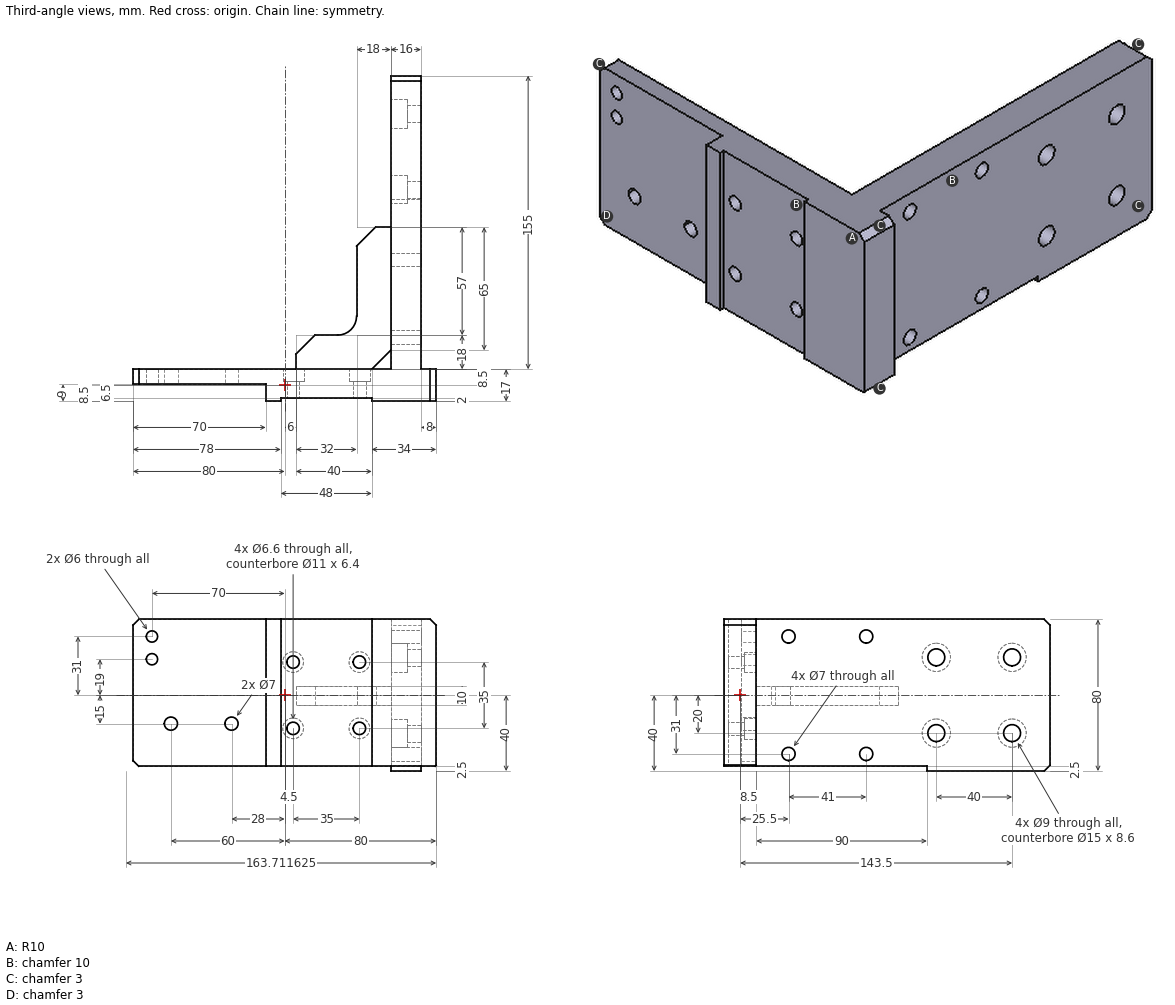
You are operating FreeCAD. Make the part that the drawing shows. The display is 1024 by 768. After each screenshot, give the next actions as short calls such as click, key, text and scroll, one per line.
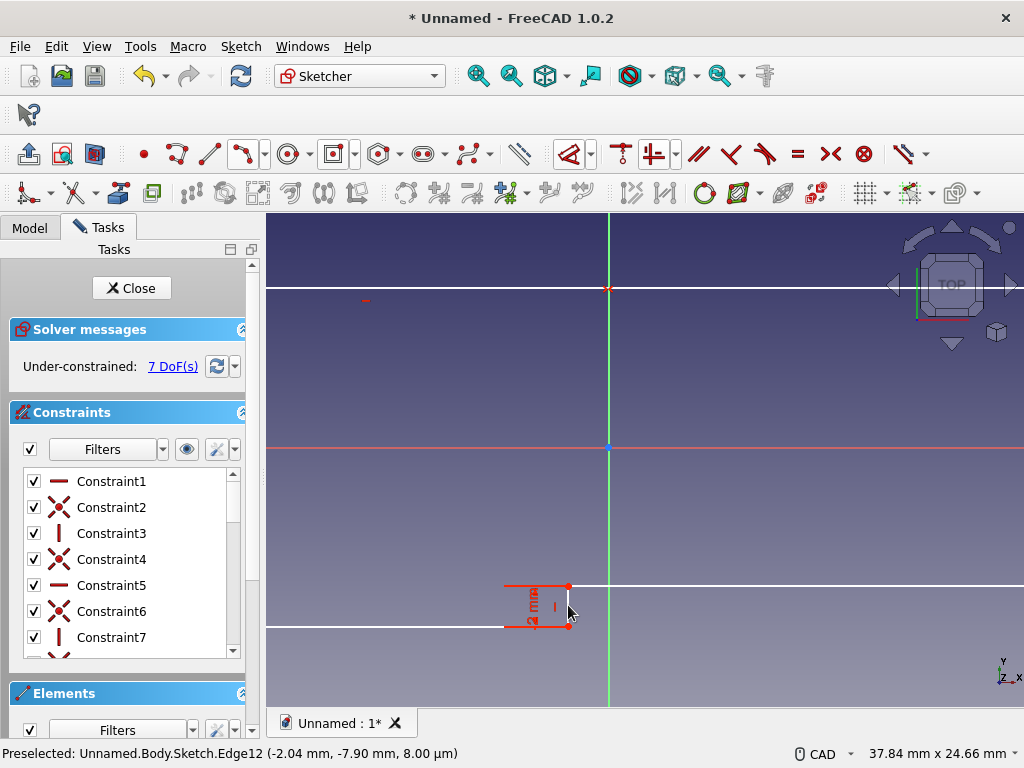
scroll(573, 616, down, 12)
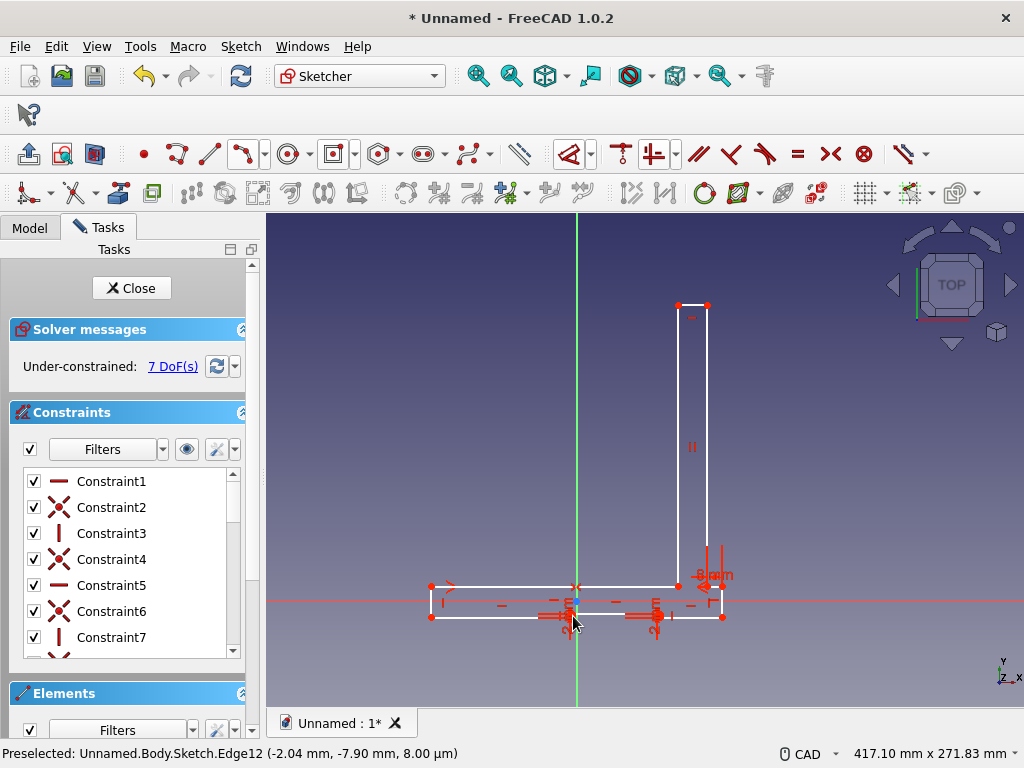
click(599, 614)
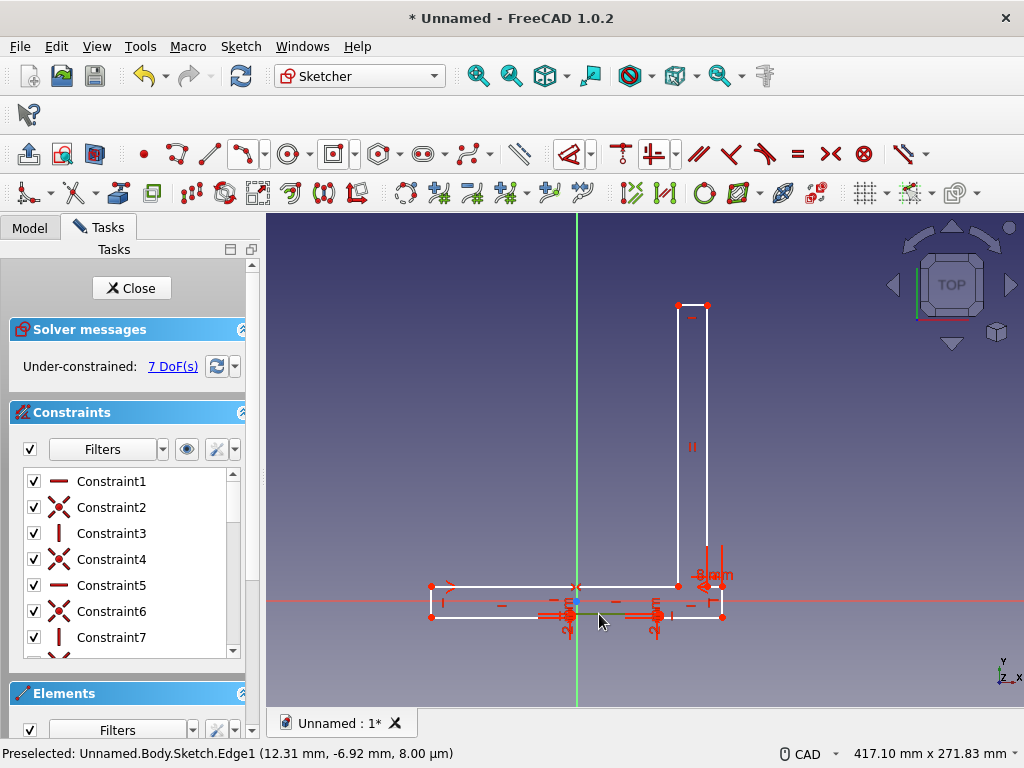
click(590, 154)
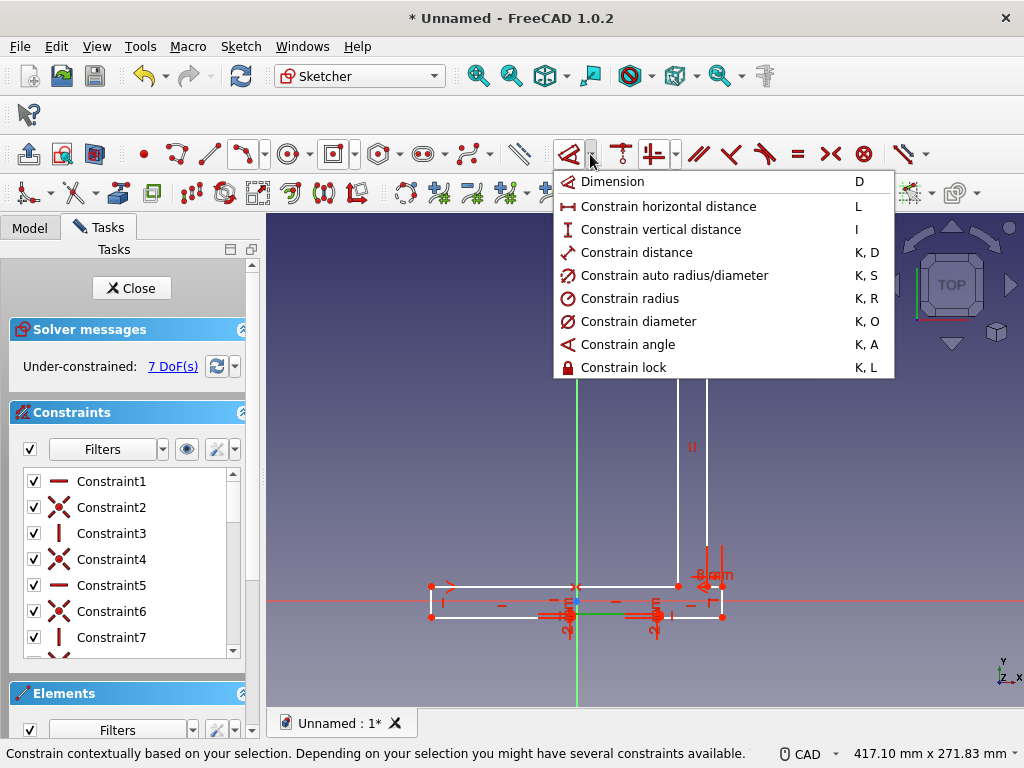
click(724, 206)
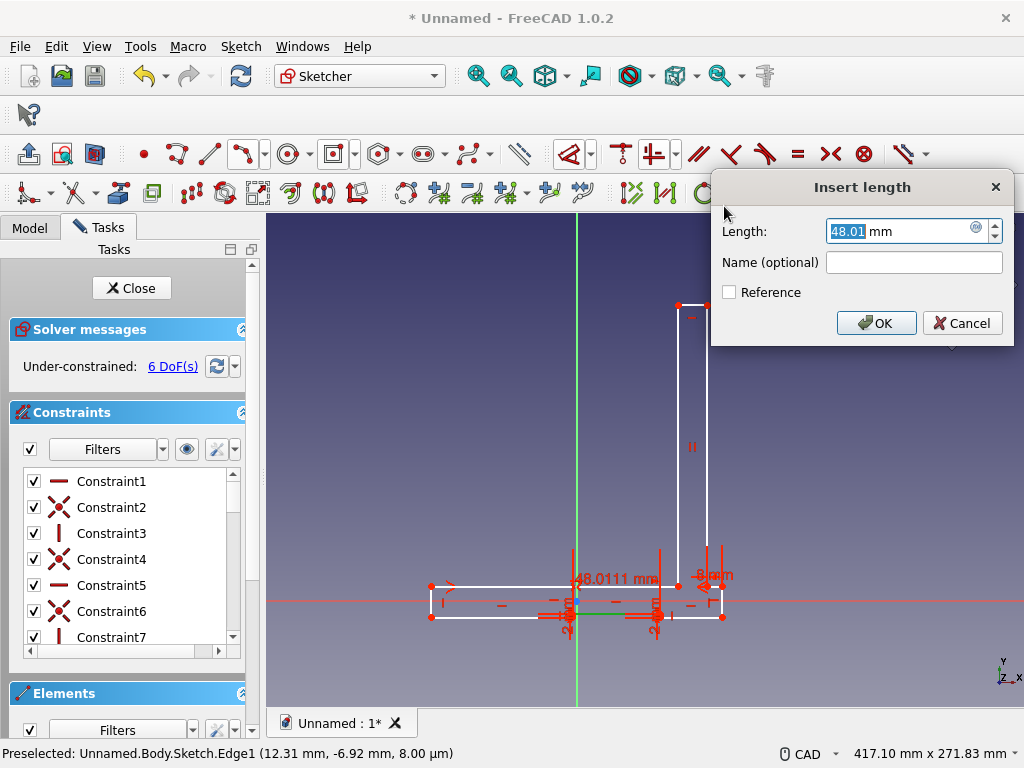
text(48)
key(Return)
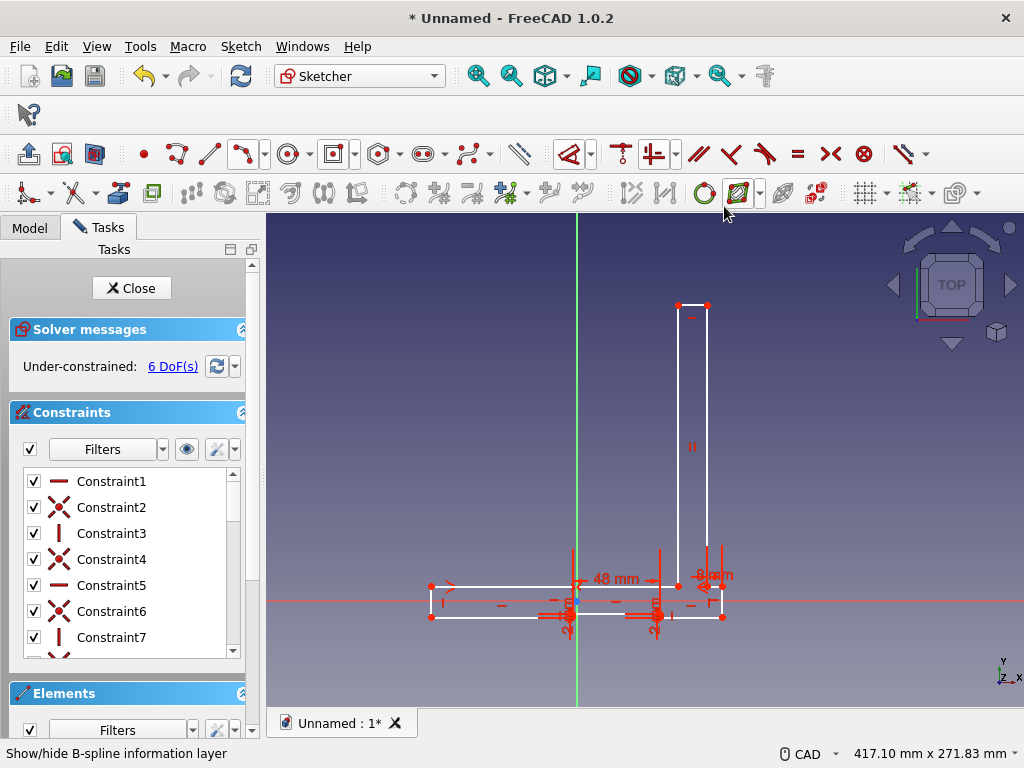
click(679, 618)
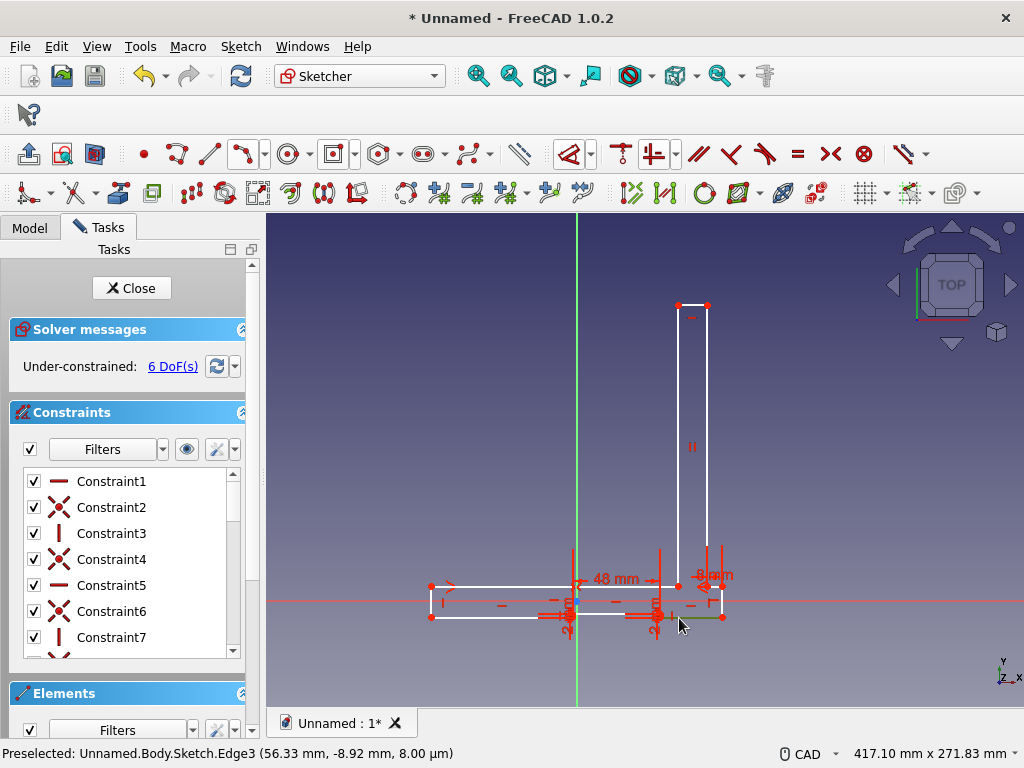
click(590, 154)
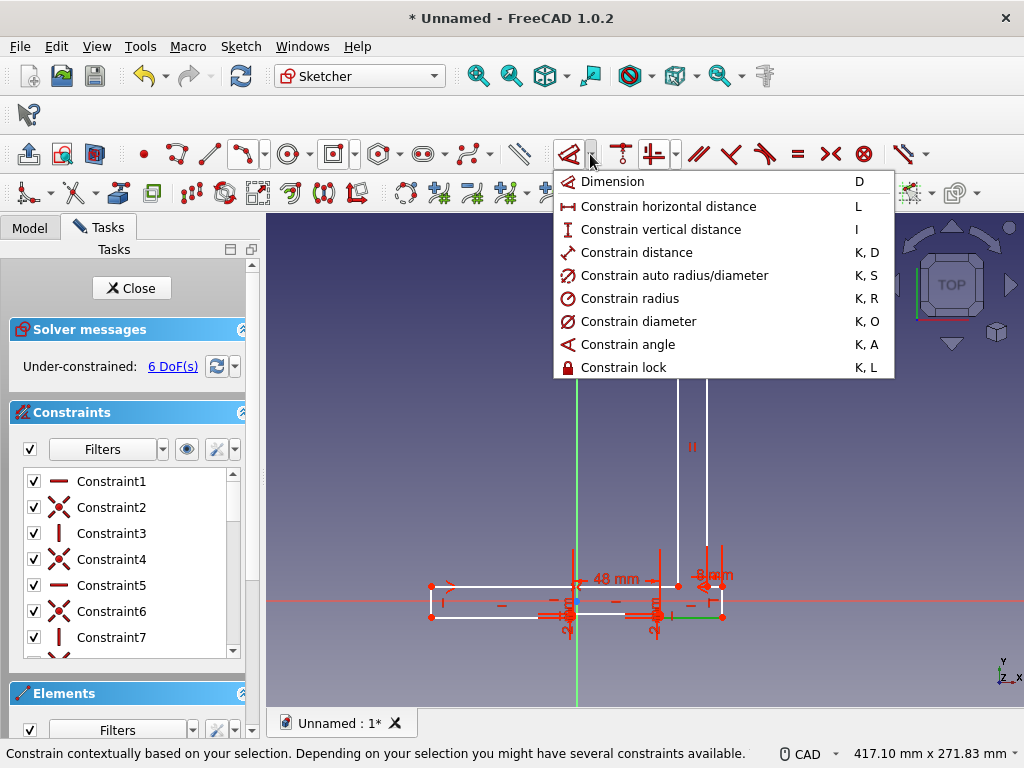
click(724, 206)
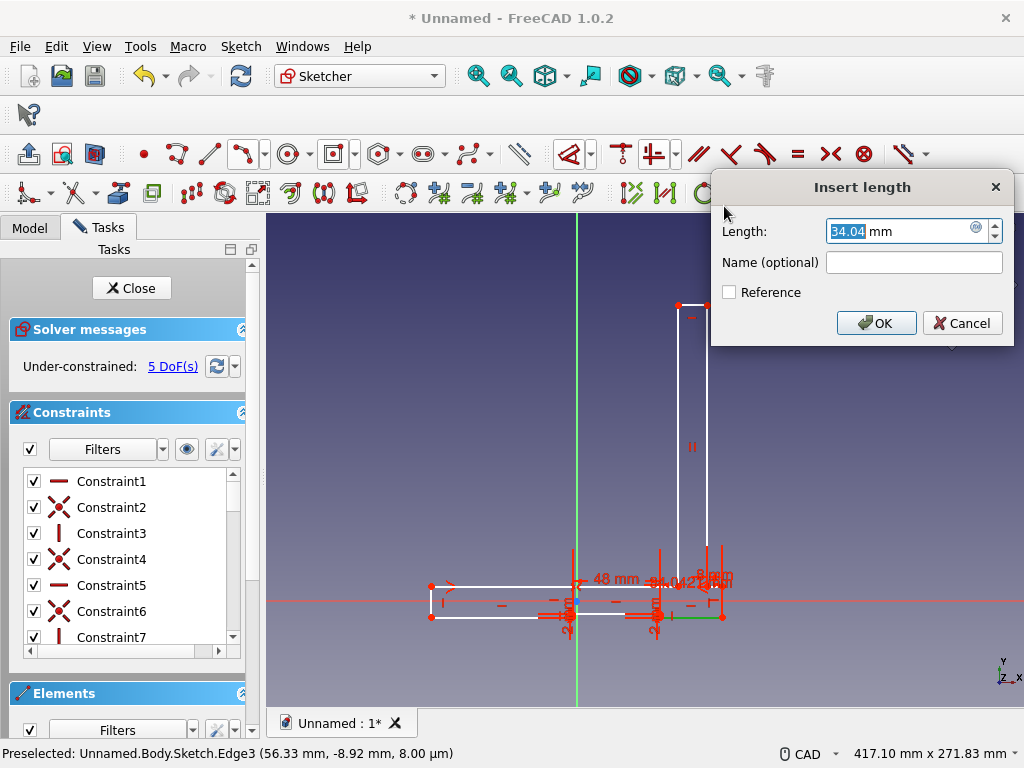
text(34)
key(Return)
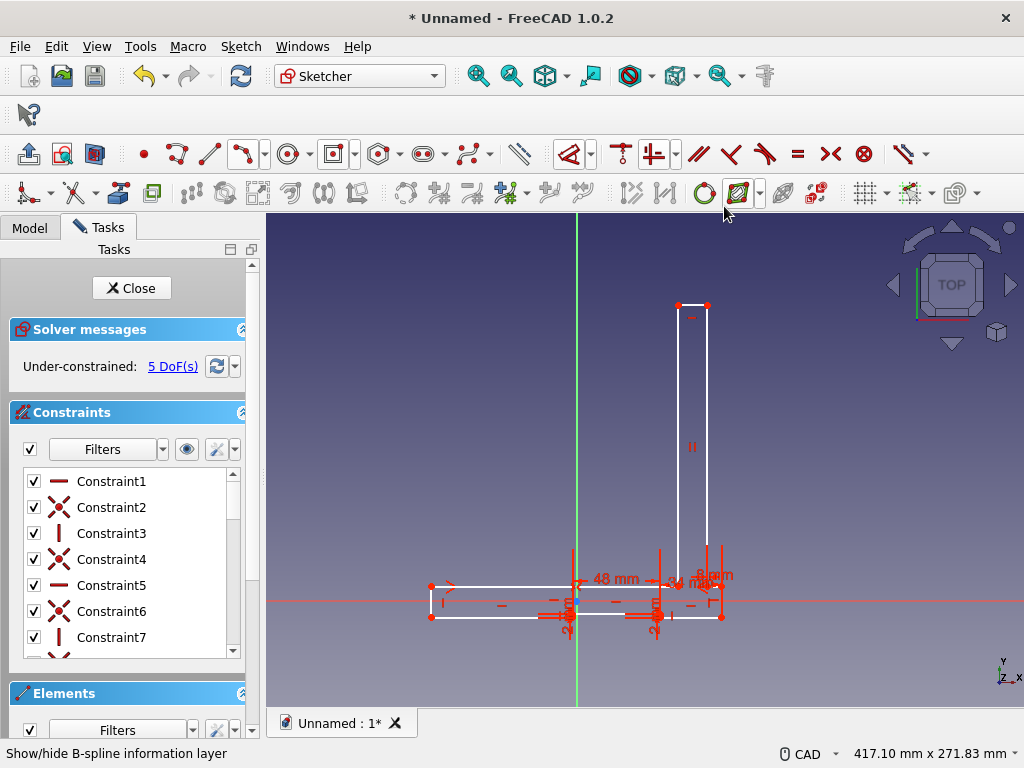
scroll(722, 605, up, 2)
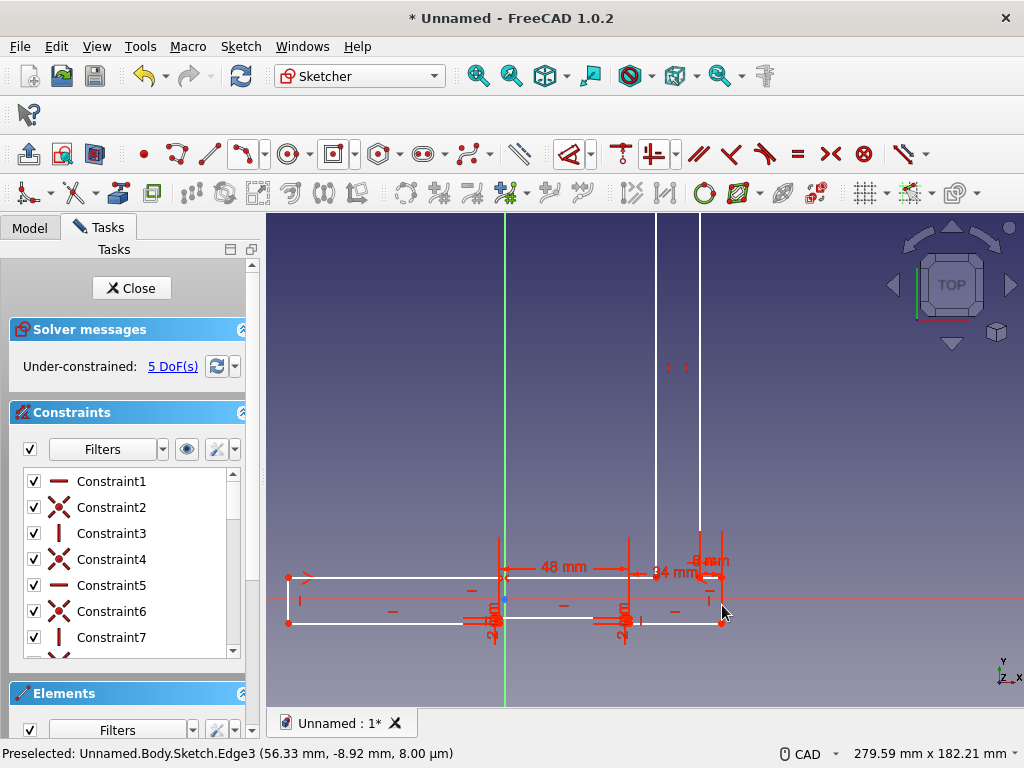
click(722, 605)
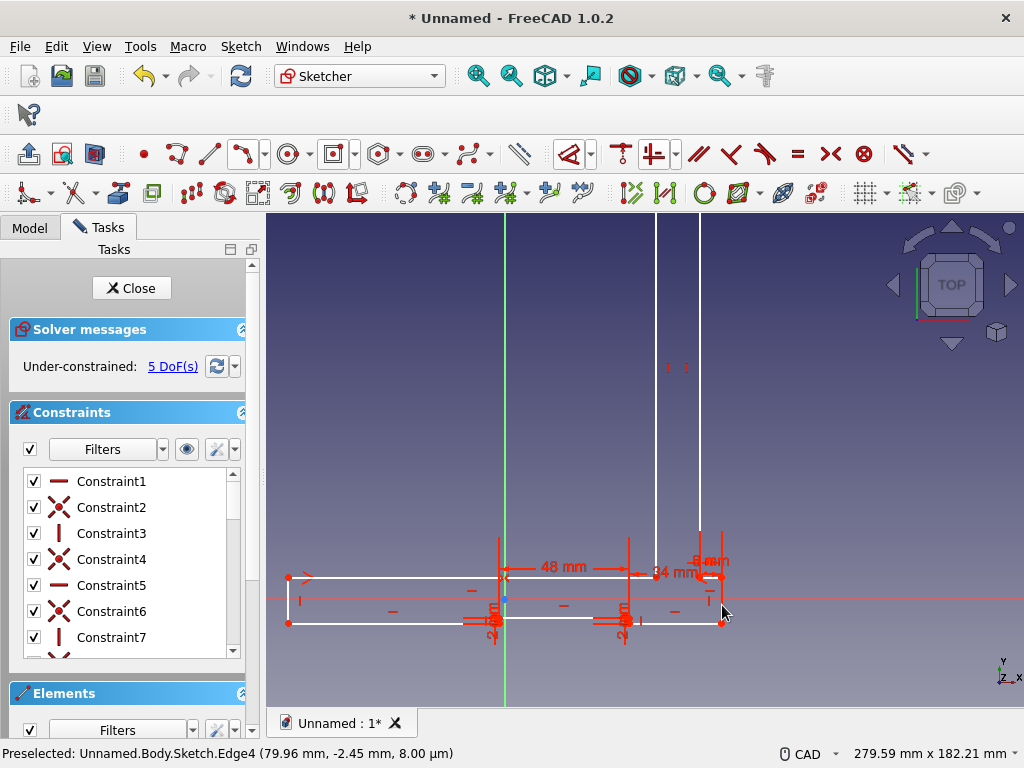
click(590, 154)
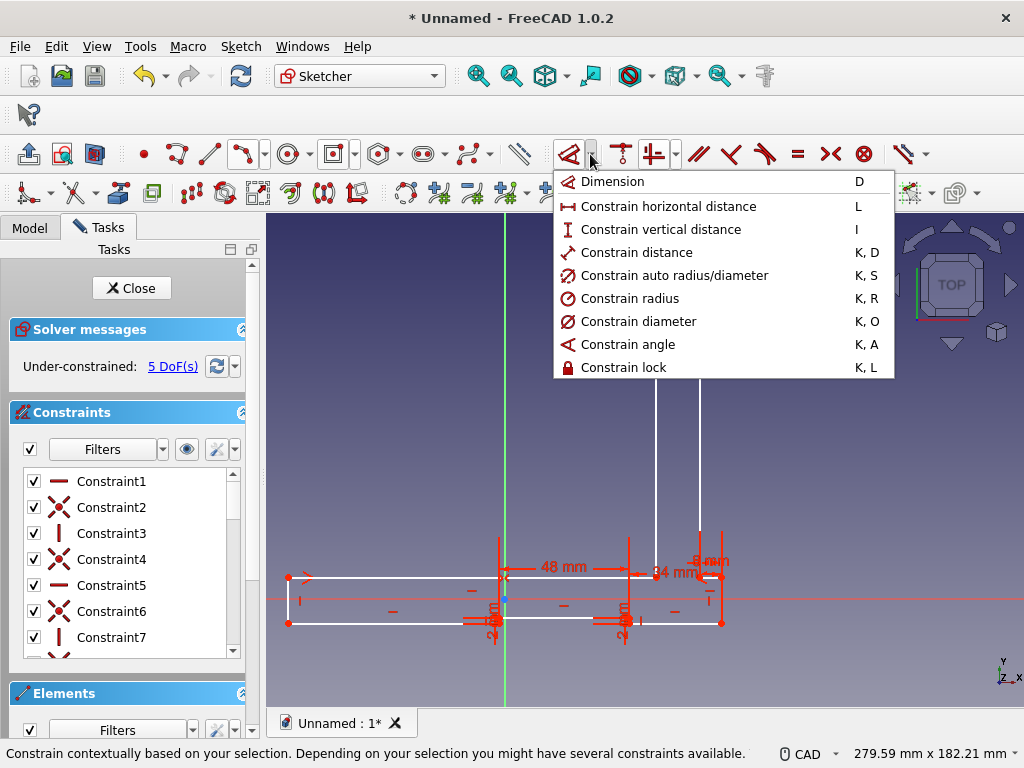
click(724, 230)